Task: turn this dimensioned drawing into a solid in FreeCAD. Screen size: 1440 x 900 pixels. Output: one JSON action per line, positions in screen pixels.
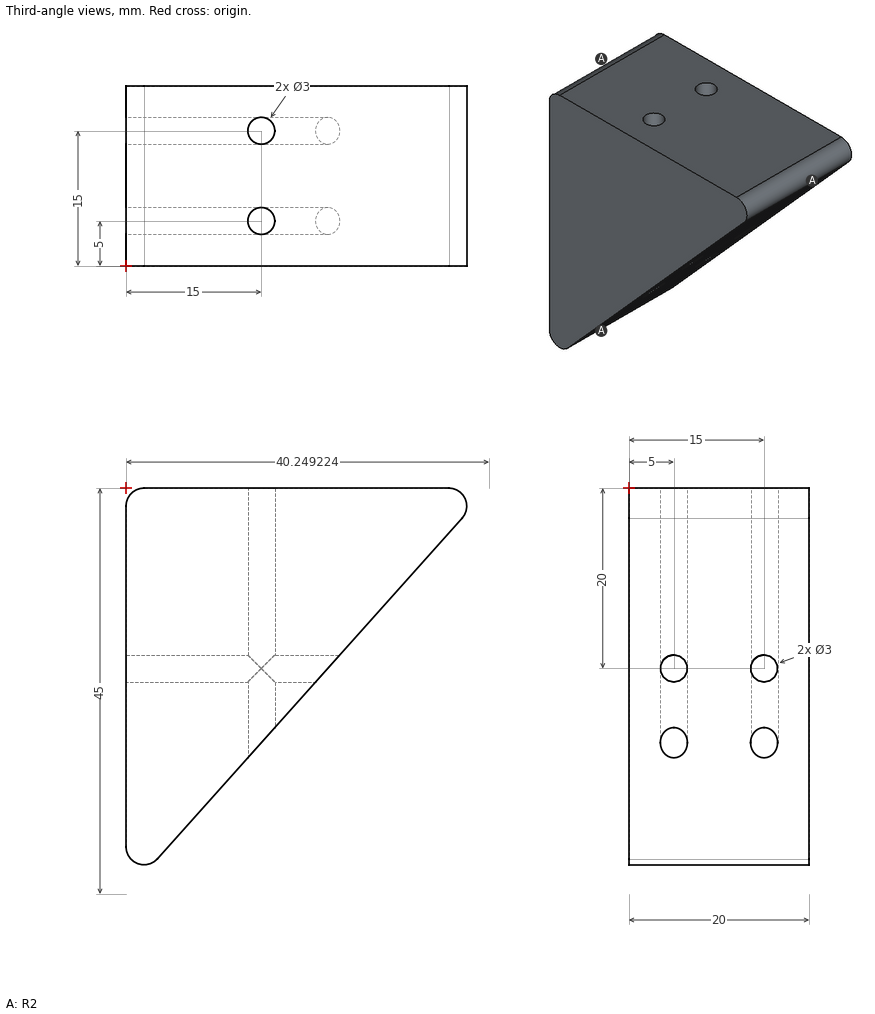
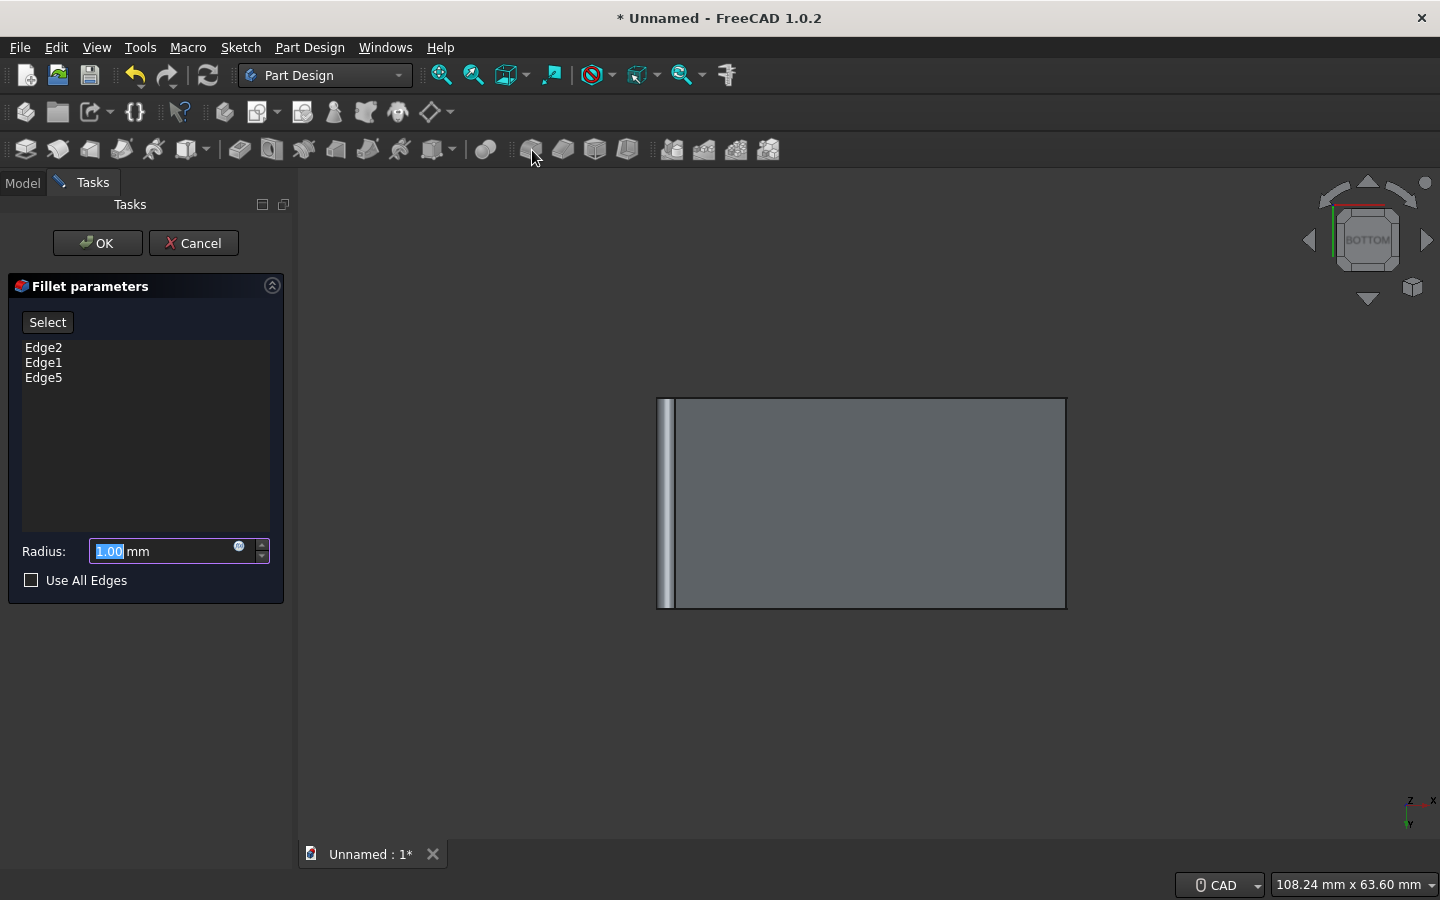
{"action": "type", "text": "2"}
{"action": "key", "text": "Tab"}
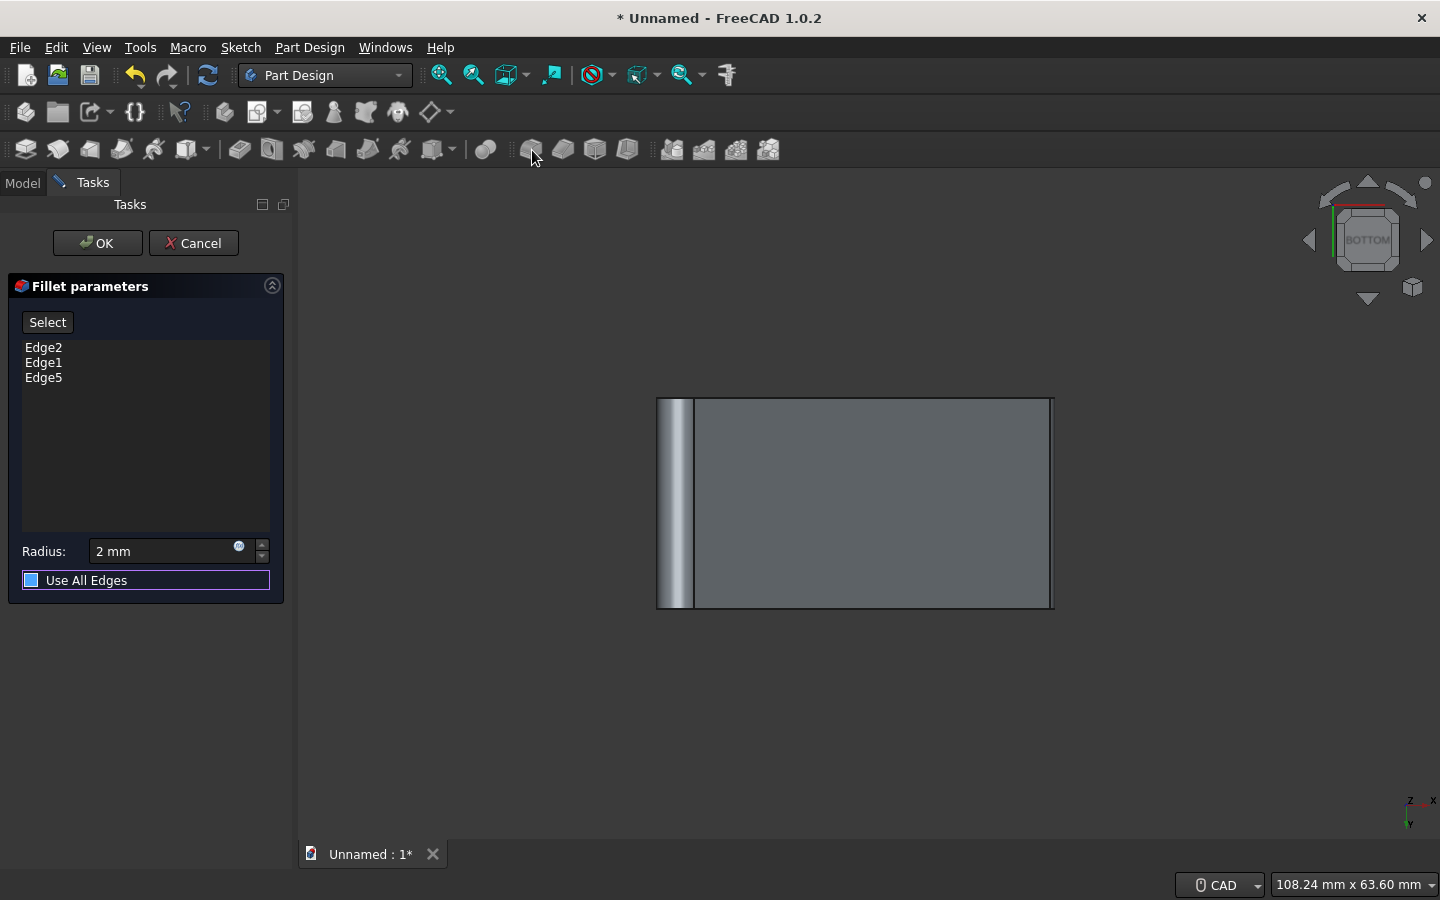
{"action": "left_click", "coordinate": [98, 243]}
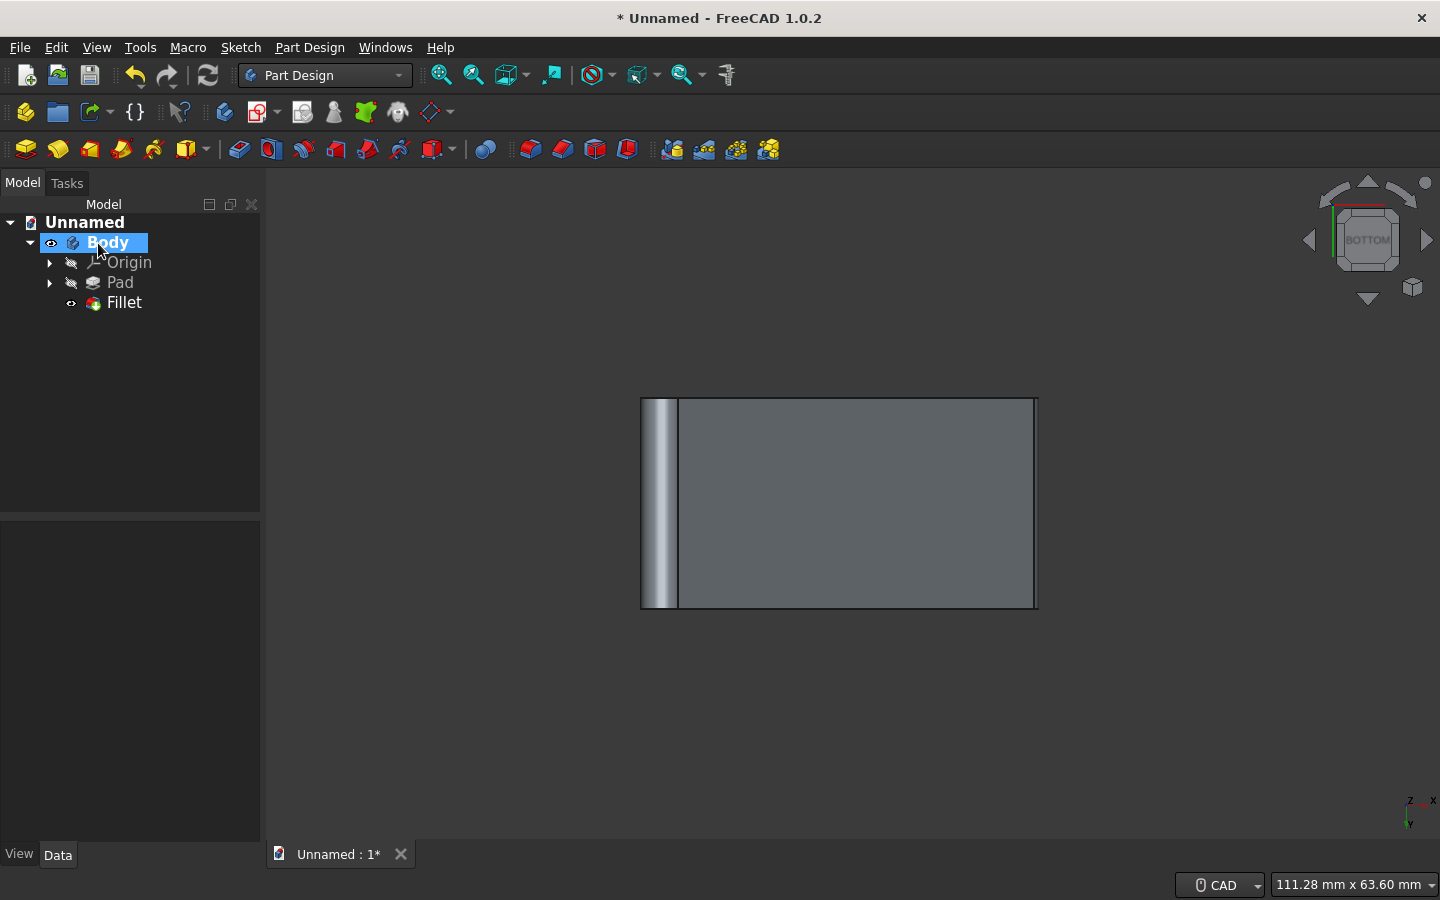
{"action": "key", "text": "v f"}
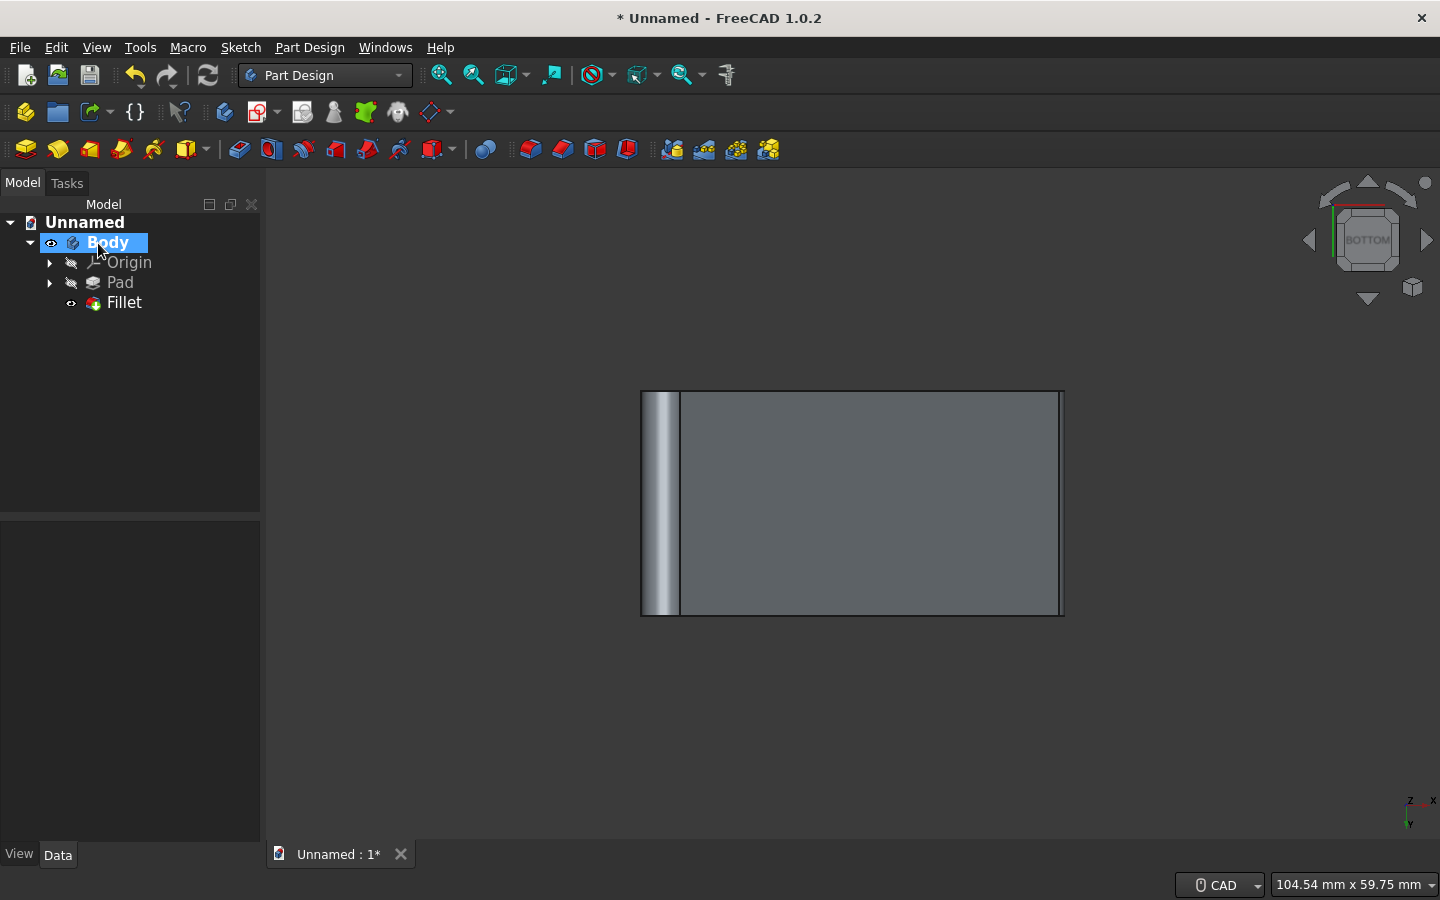
{"action": "left_click", "coordinate": [258, 112]}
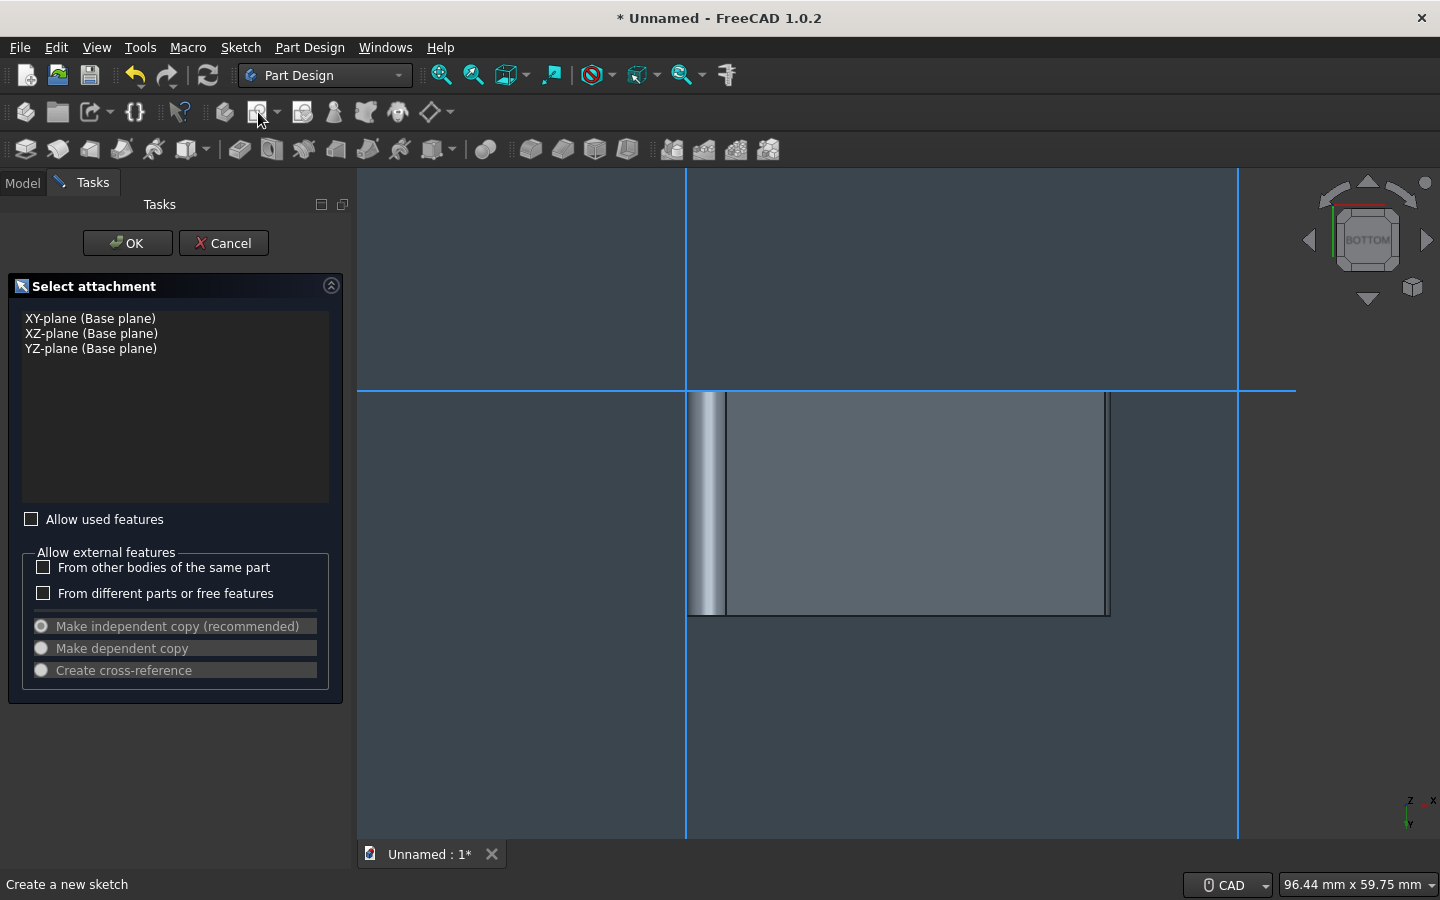
{"action": "left_click", "coordinate": [82, 348]}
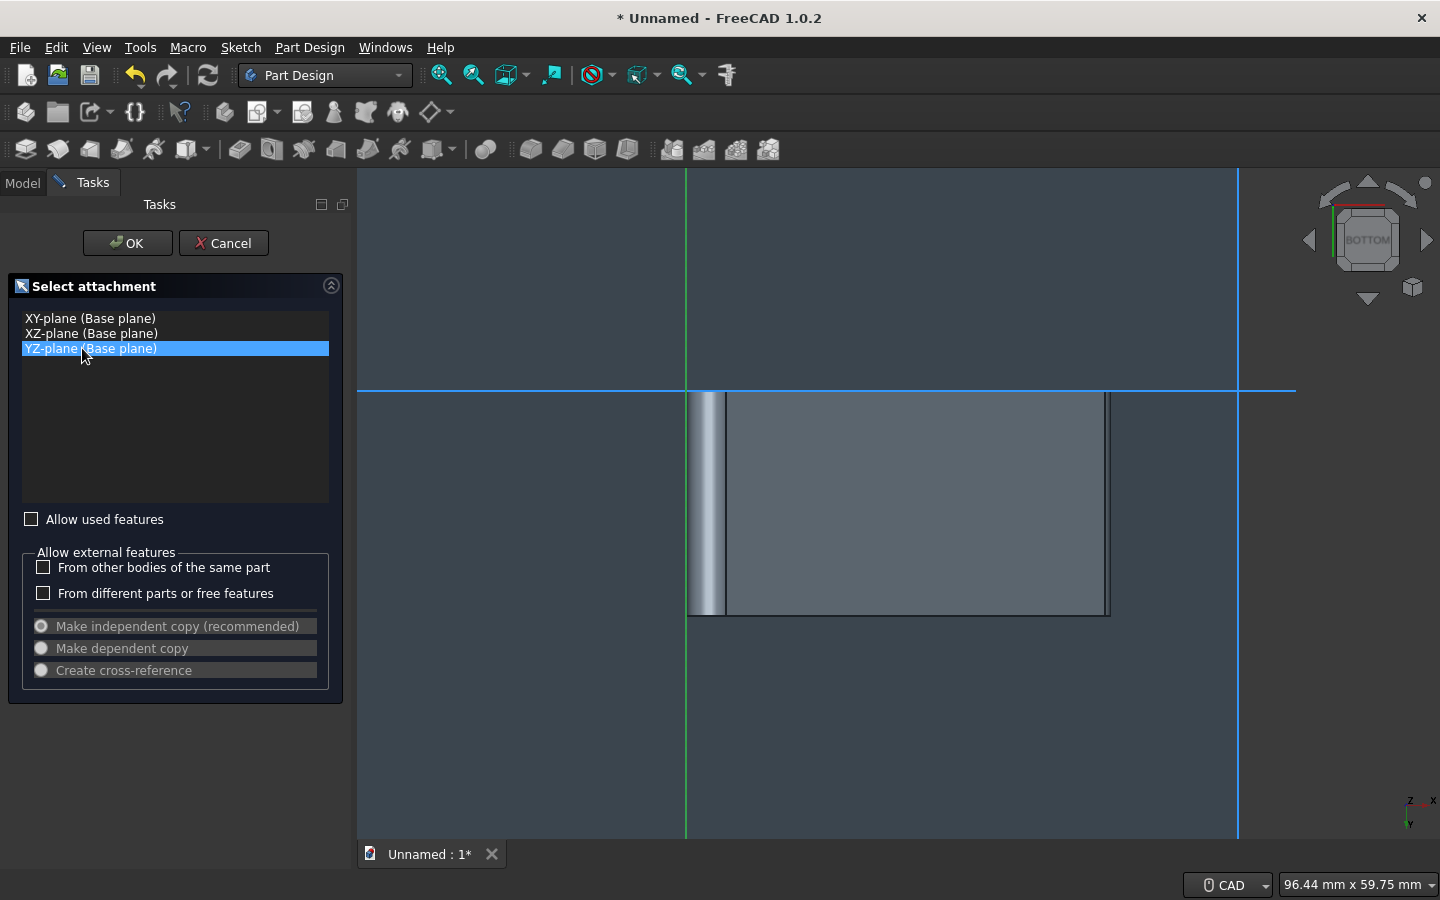
{"action": "left_click", "coordinate": [128, 243]}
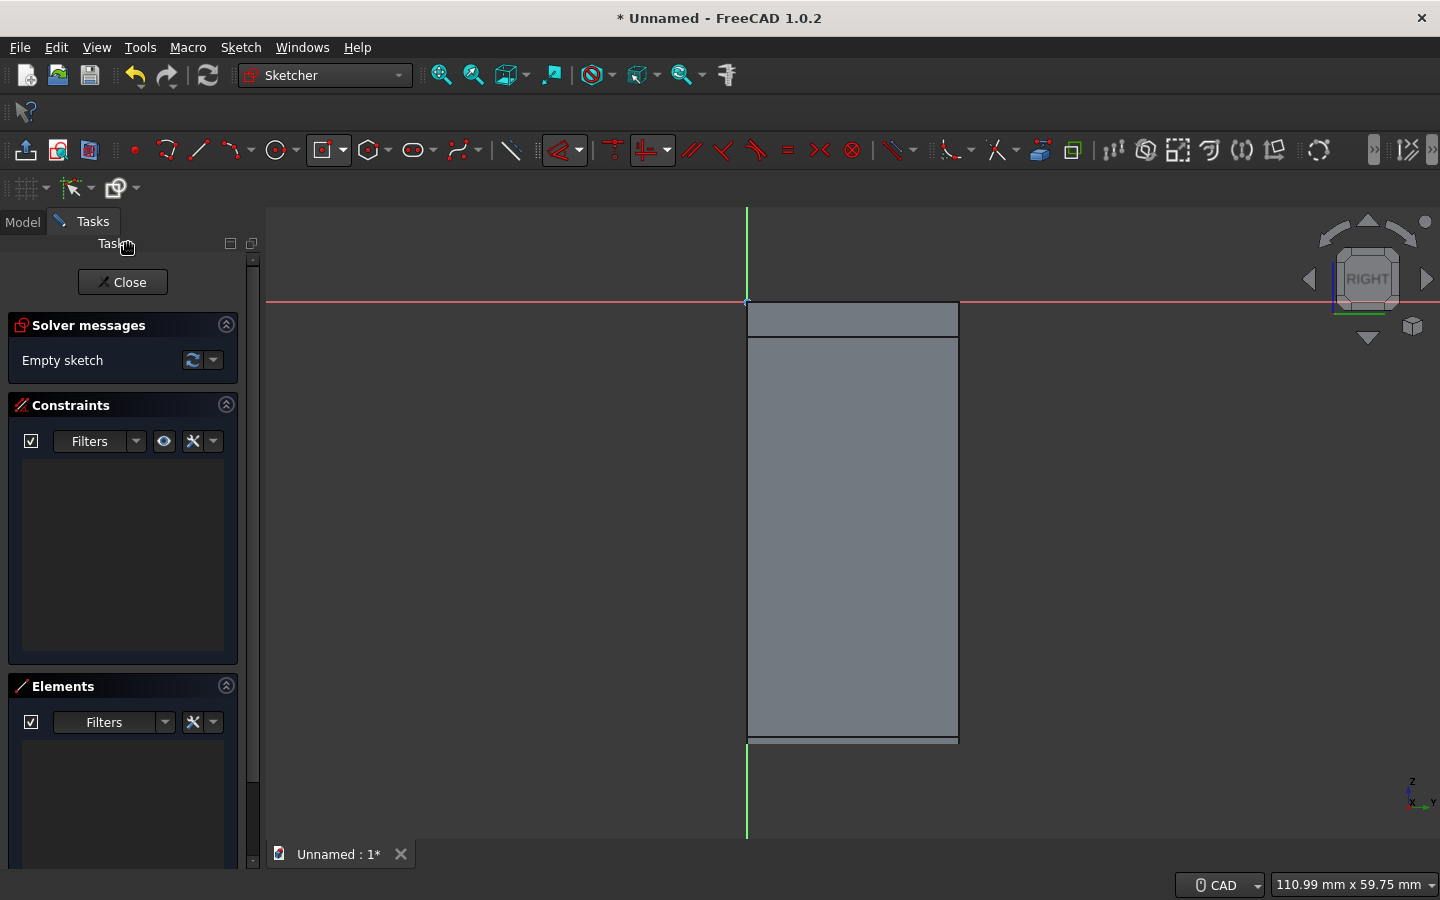
{"action": "key", "text": "q s"}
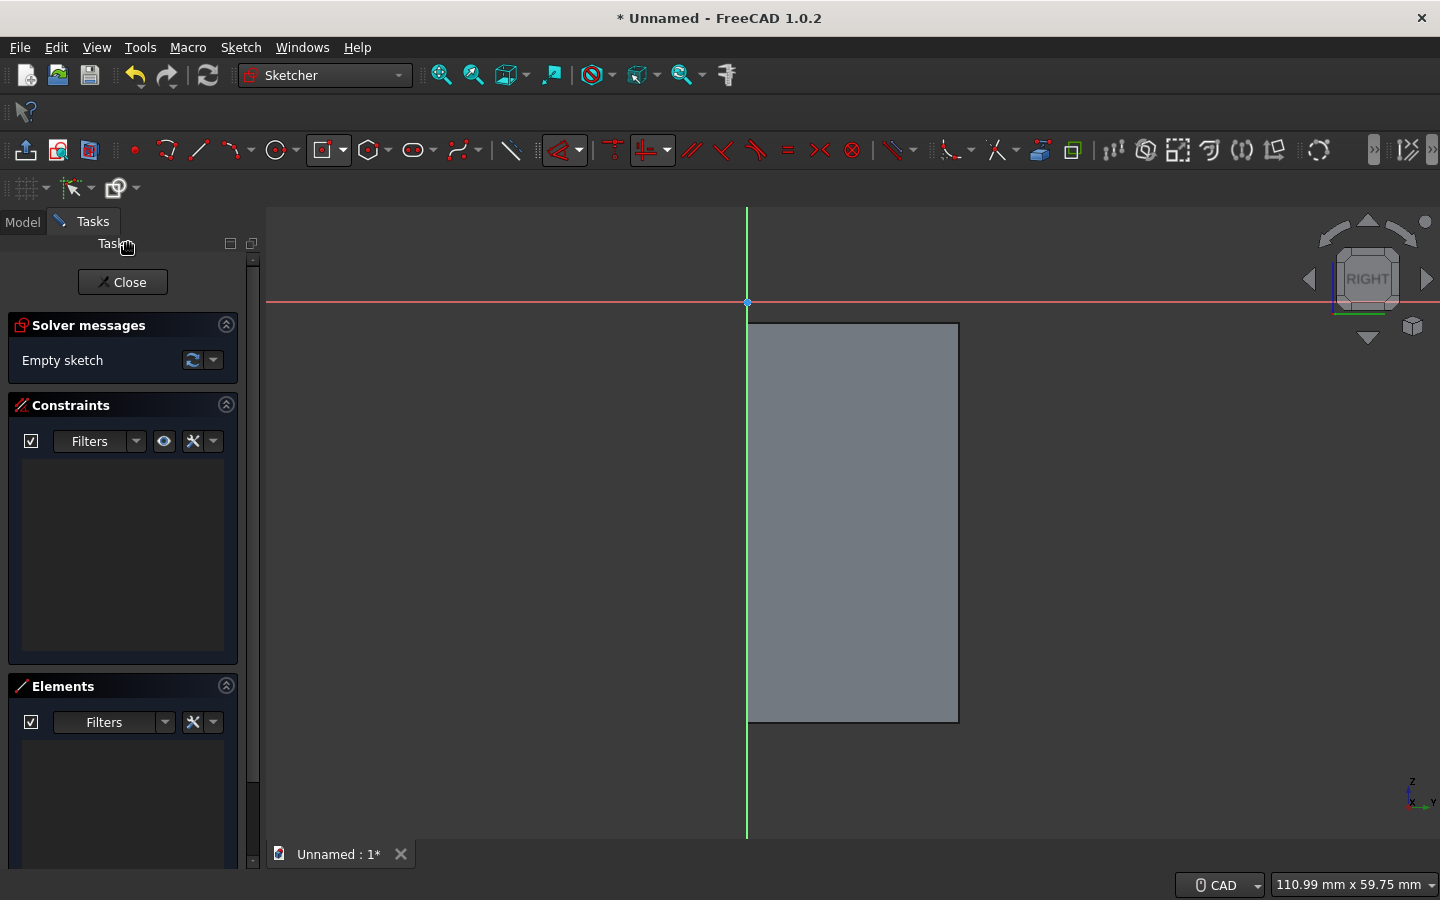
{"action": "scroll", "coordinate": [895, 286], "scroll_direction": "up", "scroll_amount": 3}